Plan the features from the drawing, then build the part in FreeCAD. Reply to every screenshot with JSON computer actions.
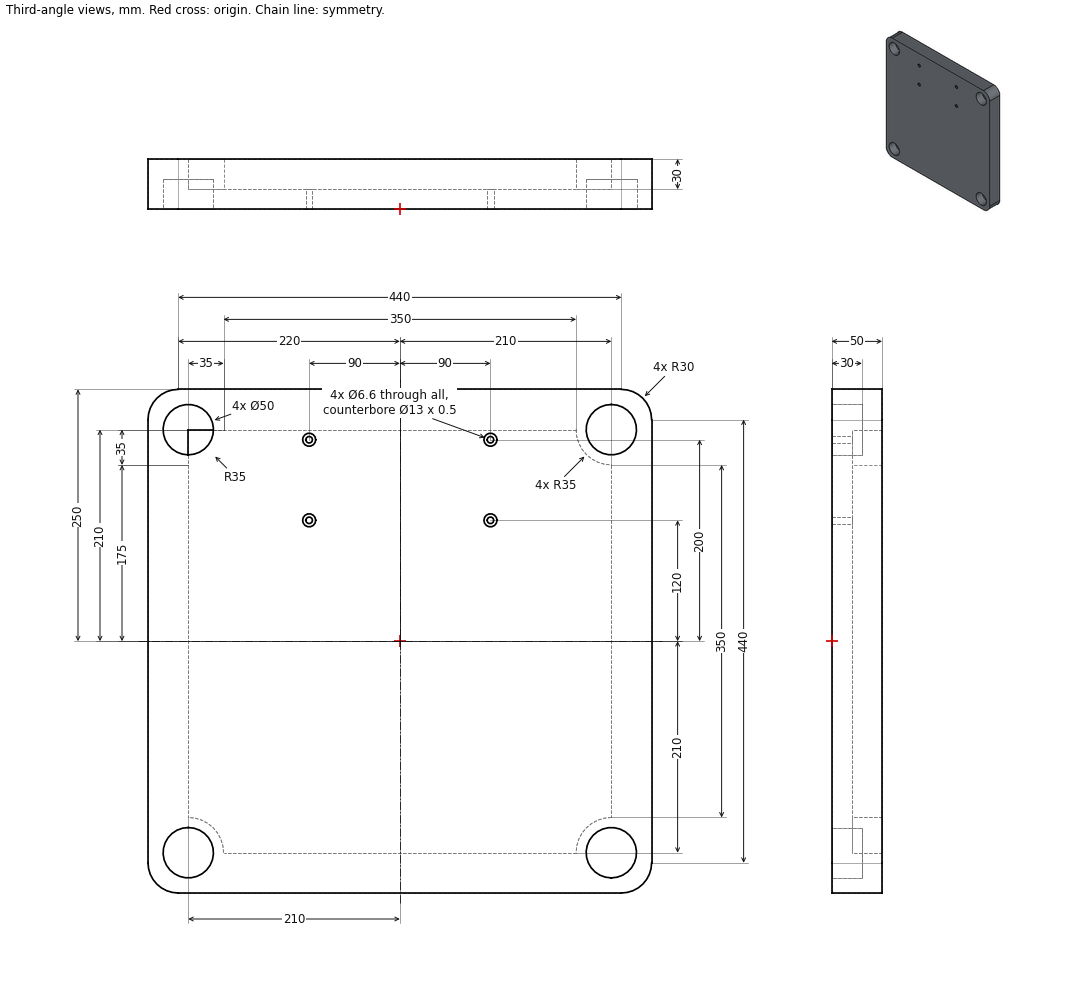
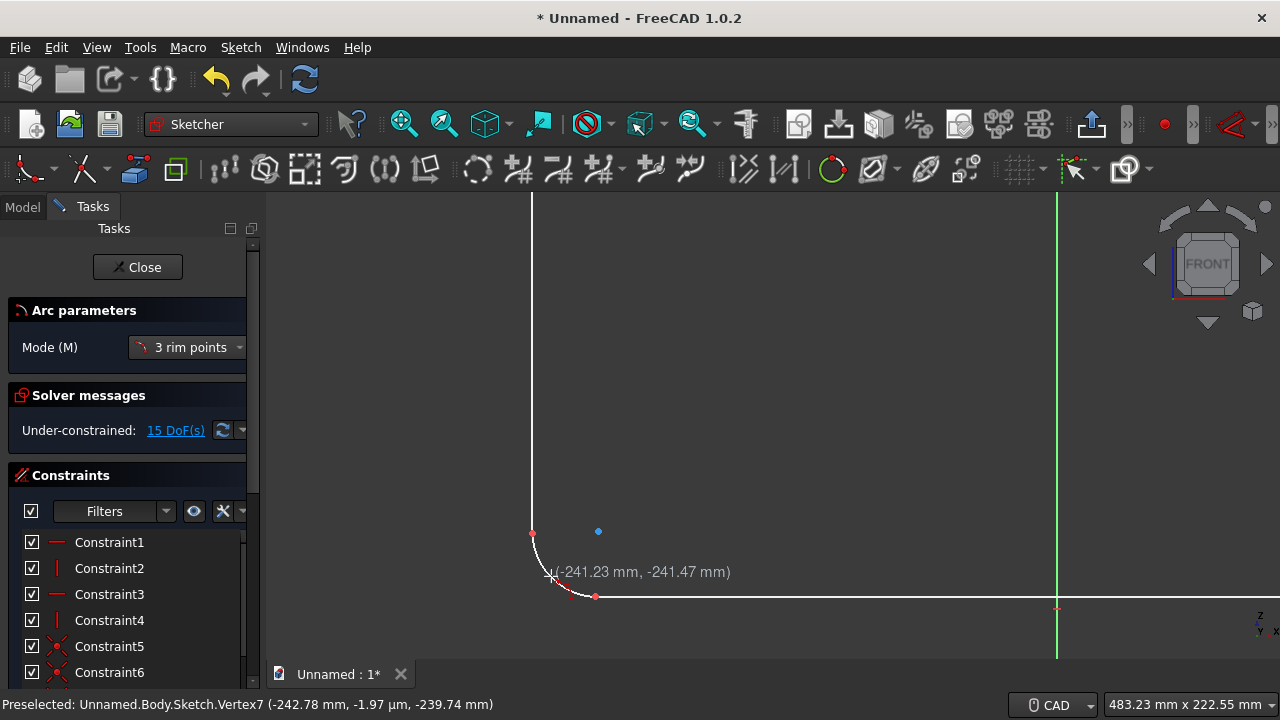
{"action": "scroll", "coordinate": [552, 579], "scroll_direction": "down", "scroll_amount": 6}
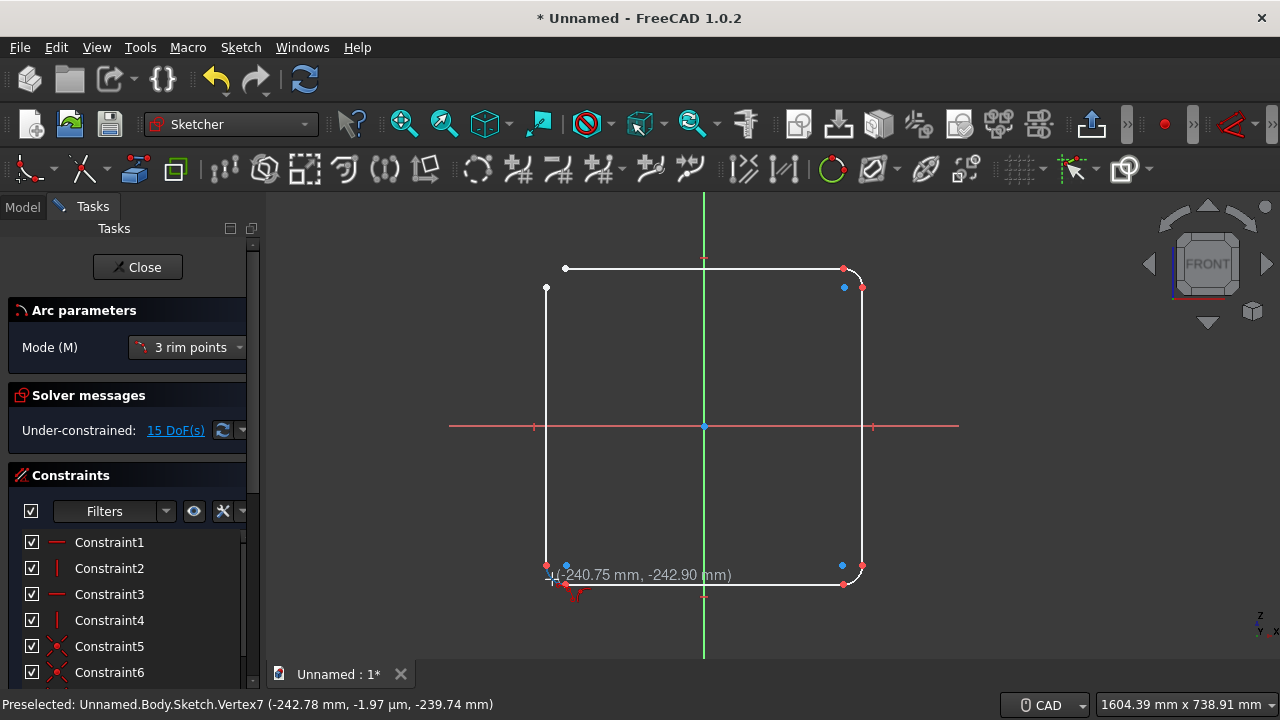
{"action": "left_click", "coordinate": [546, 288]}
{"action": "left_click", "coordinate": [565, 269]}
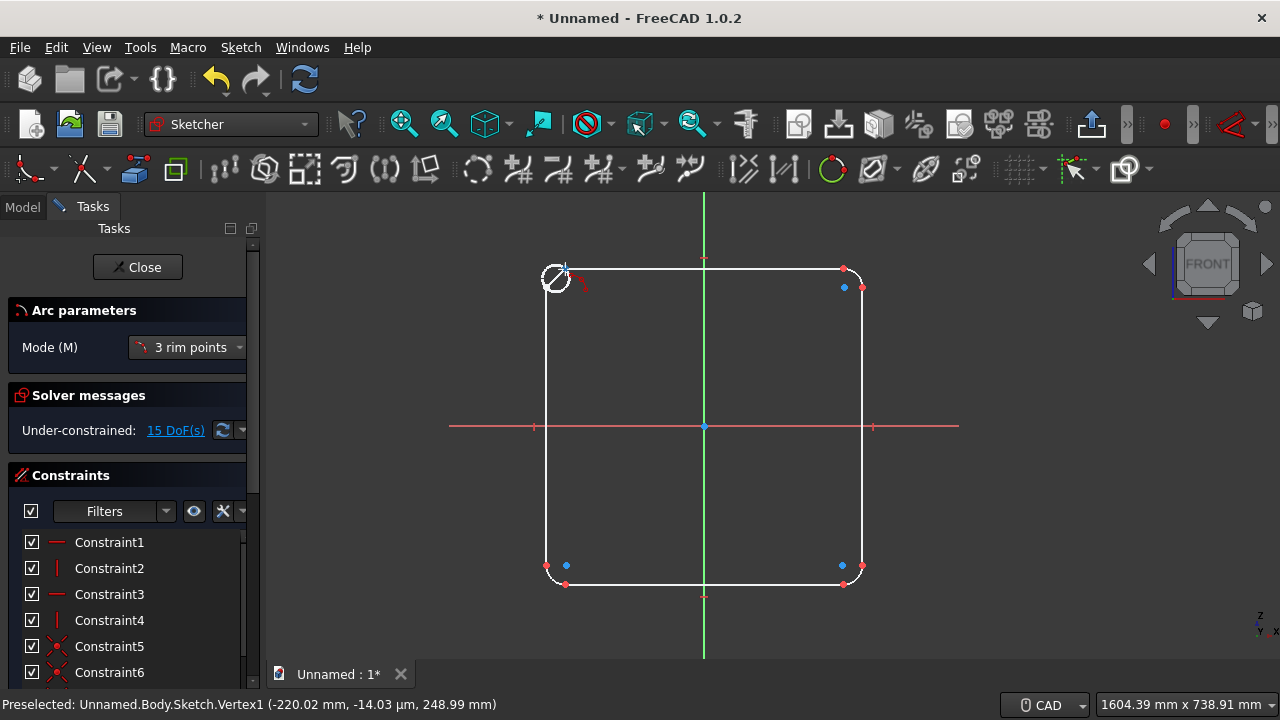
{"action": "scroll", "coordinate": [552, 274], "scroll_direction": "up", "scroll_amount": 6}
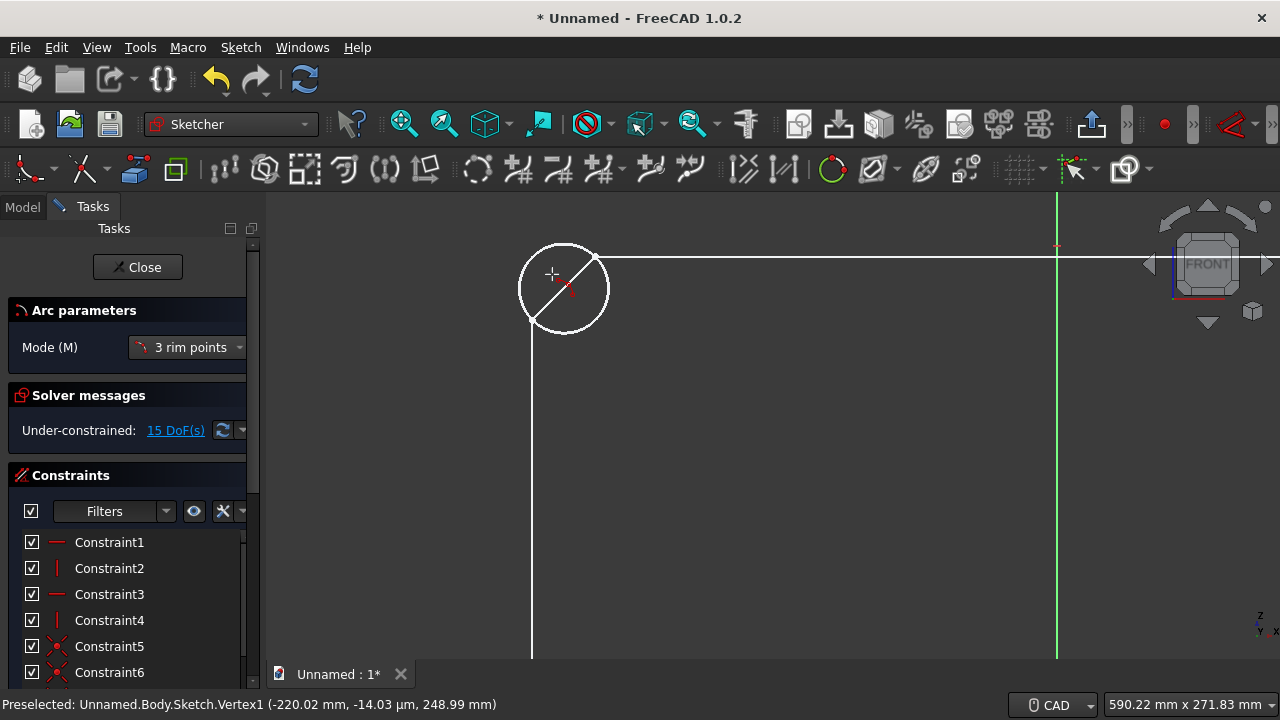
{"action": "left_click", "coordinate": [551, 273]}
{"action": "key", "text": "Escape"}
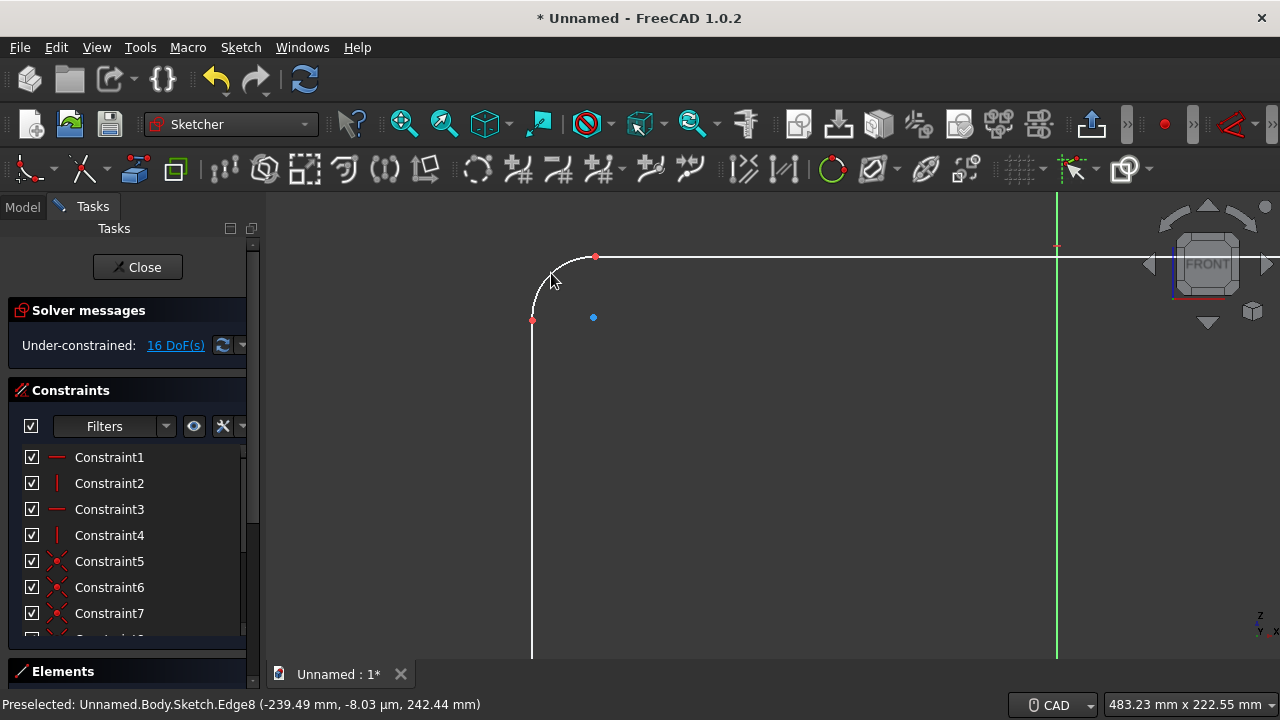
{"action": "left_click", "coordinate": [872, 257]}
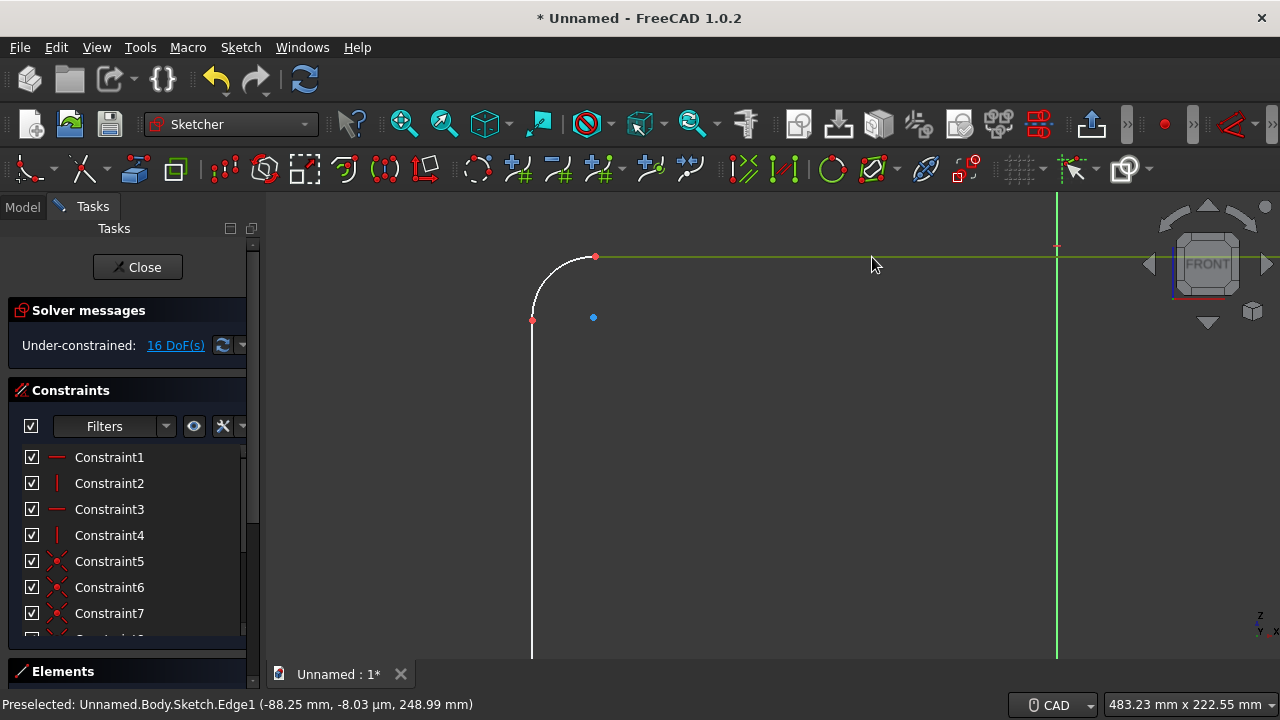
{"action": "scroll", "coordinate": [552, 273], "scroll_direction": "down", "scroll_amount": 6}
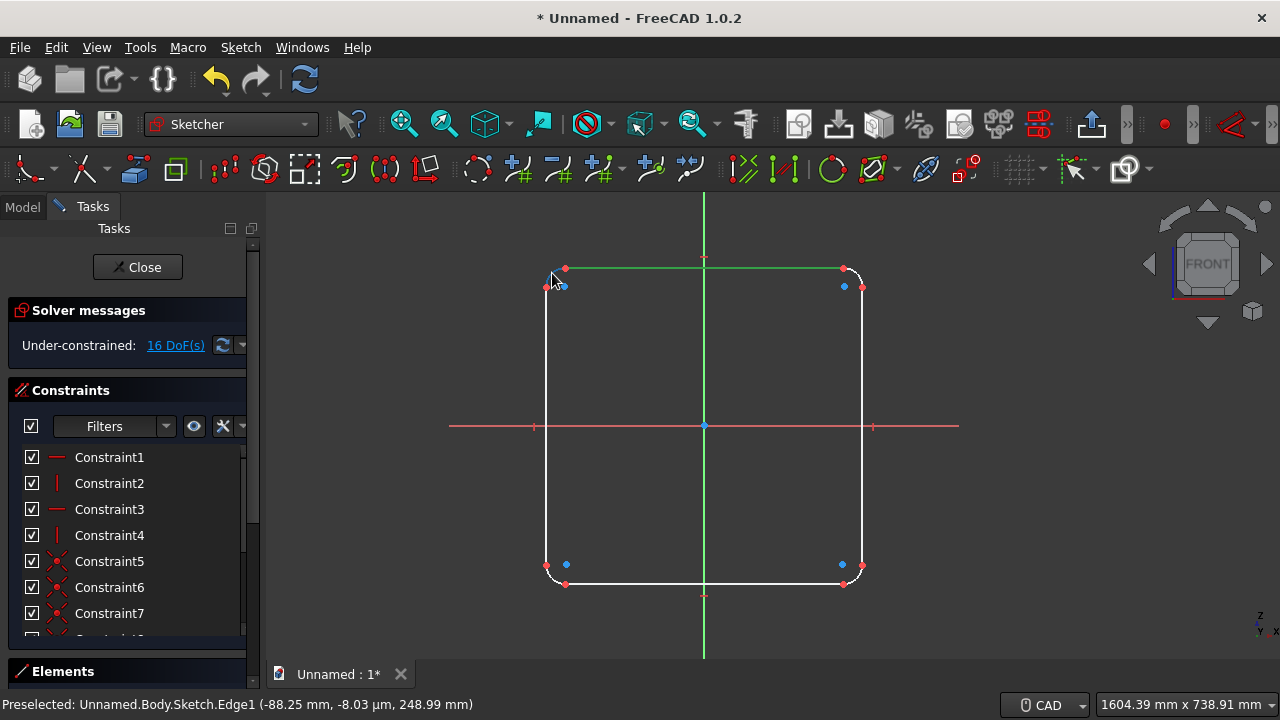
{"action": "scroll", "coordinate": [860, 279], "scroll_direction": "up", "scroll_amount": 3}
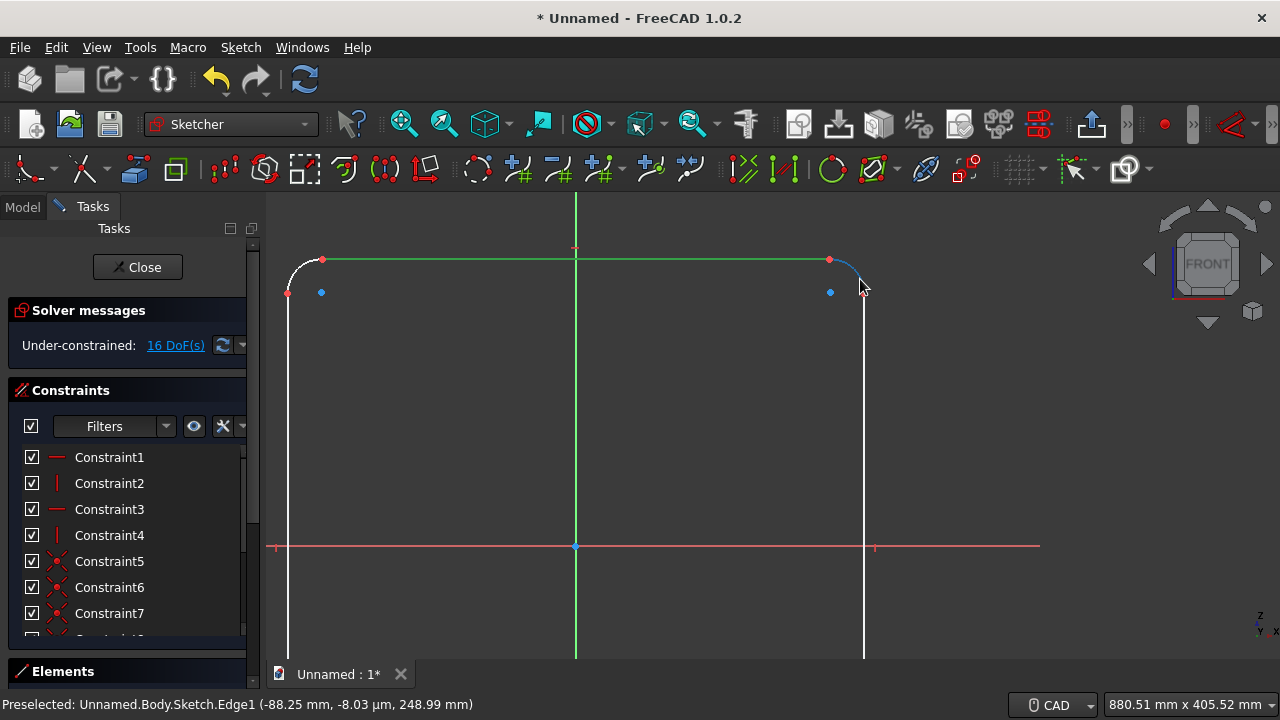
{"action": "left_click", "coordinate": [860, 278]}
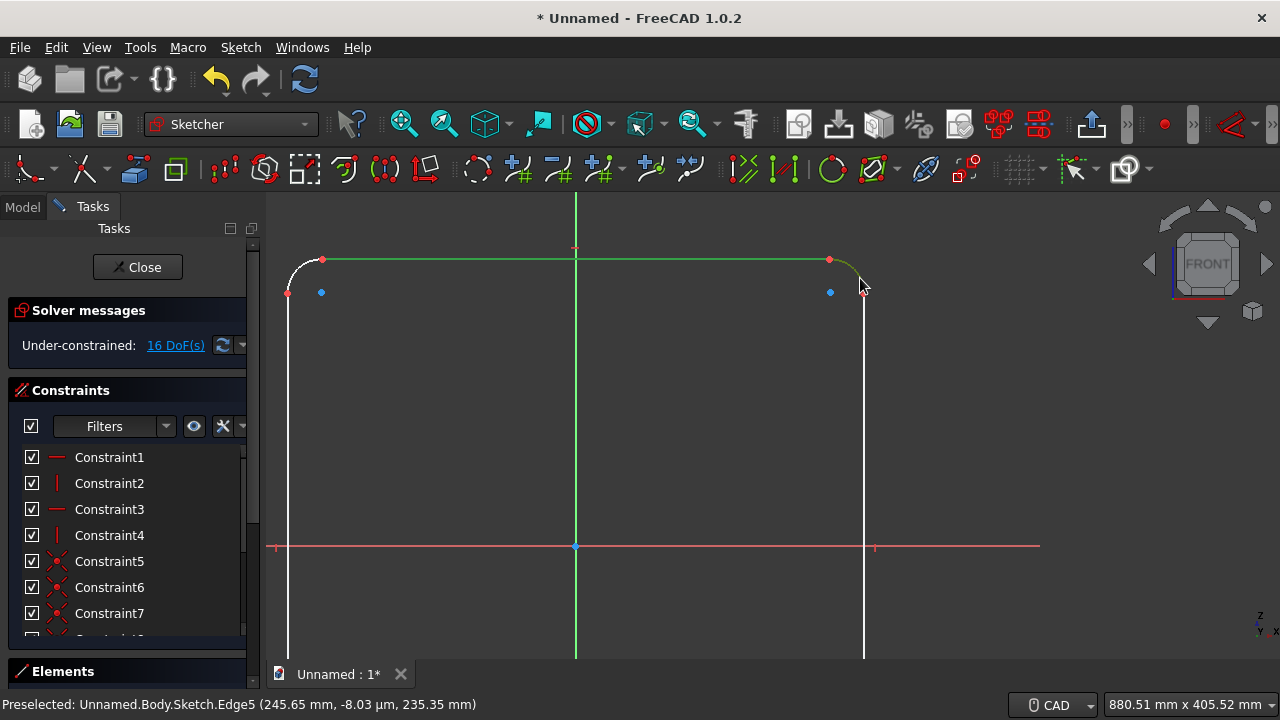
{"action": "key", "text": "t"}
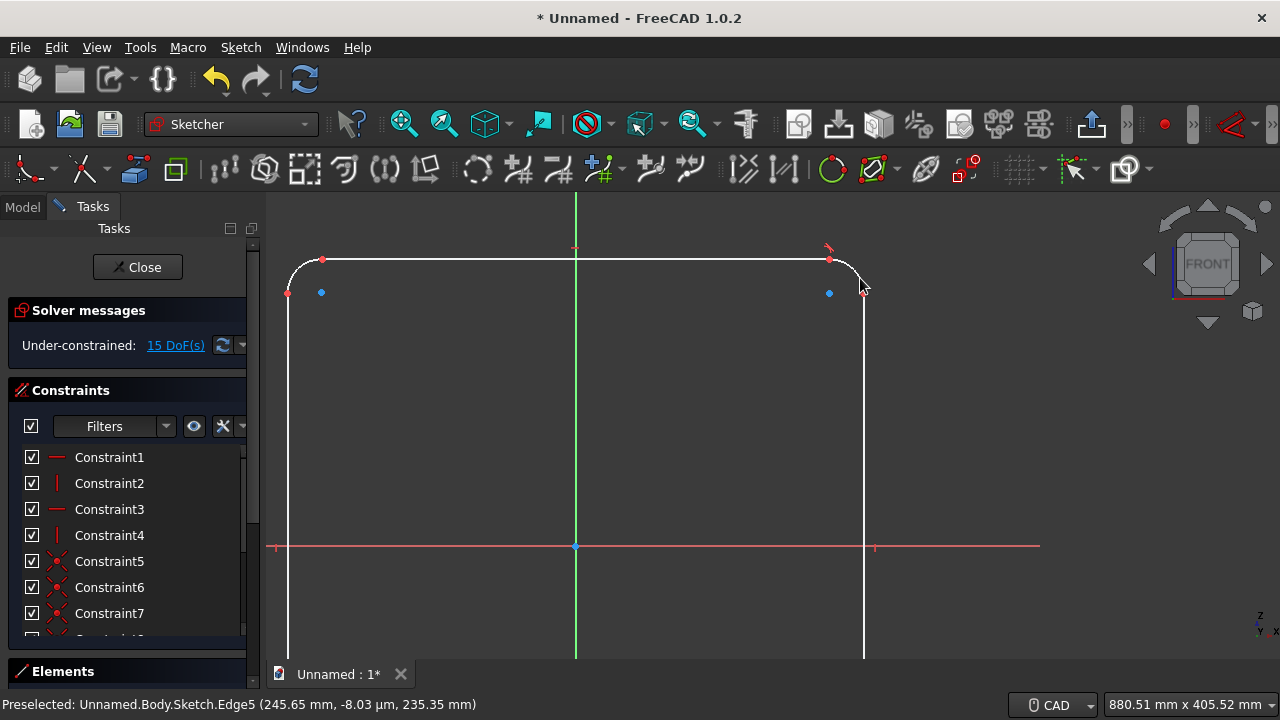
{"action": "left_click", "coordinate": [475, 259]}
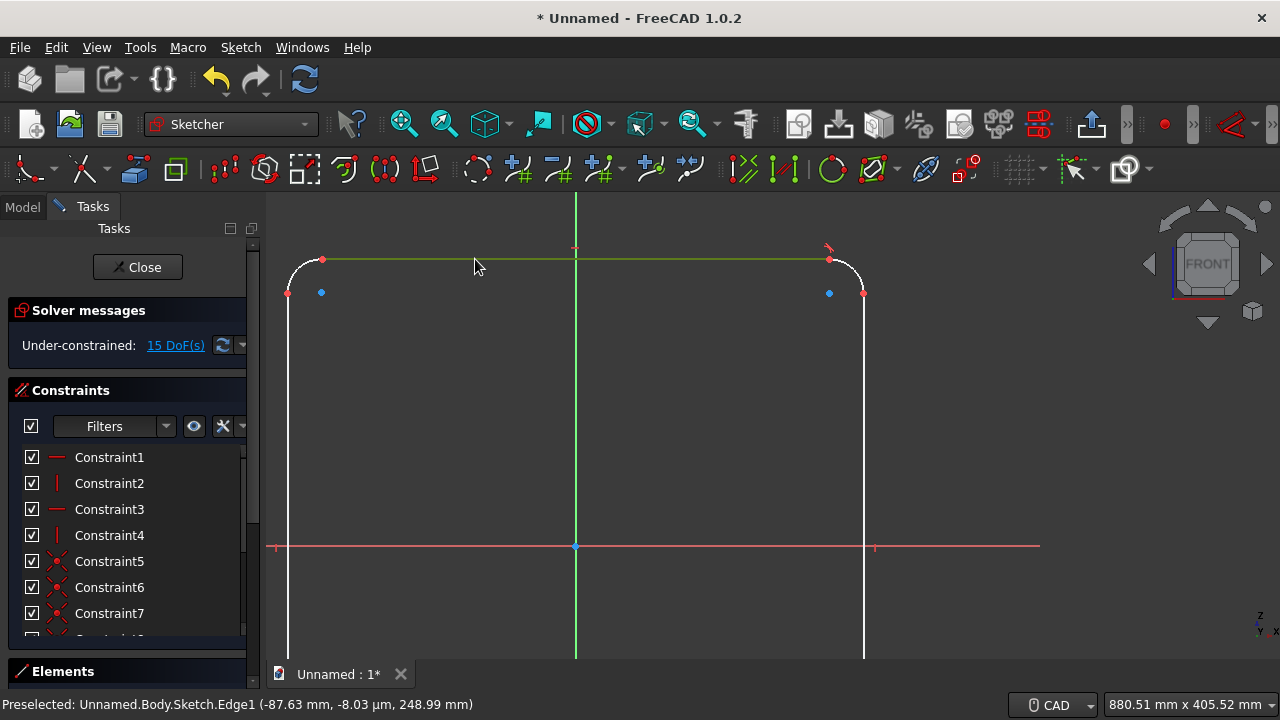
{"action": "left_click", "coordinate": [307, 263]}